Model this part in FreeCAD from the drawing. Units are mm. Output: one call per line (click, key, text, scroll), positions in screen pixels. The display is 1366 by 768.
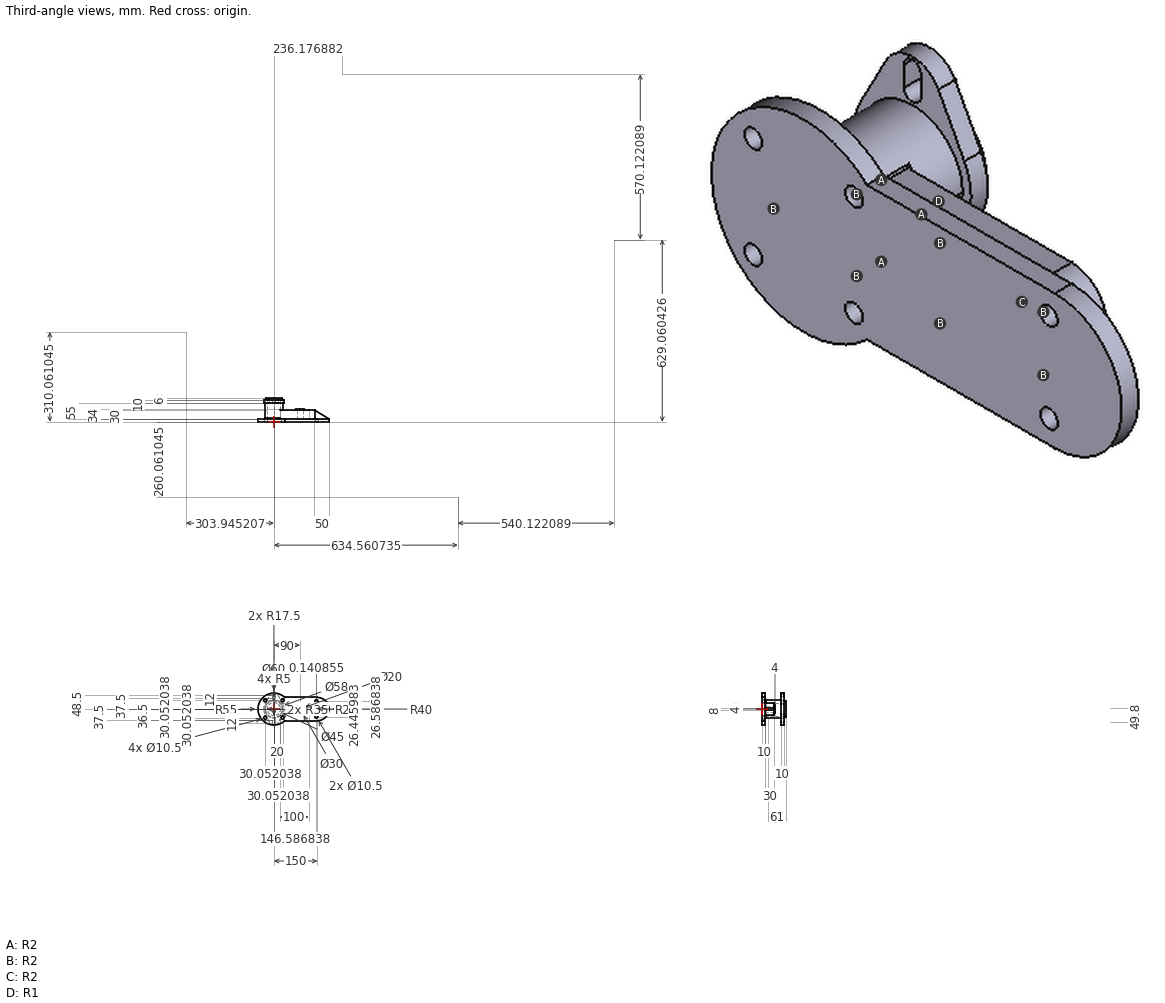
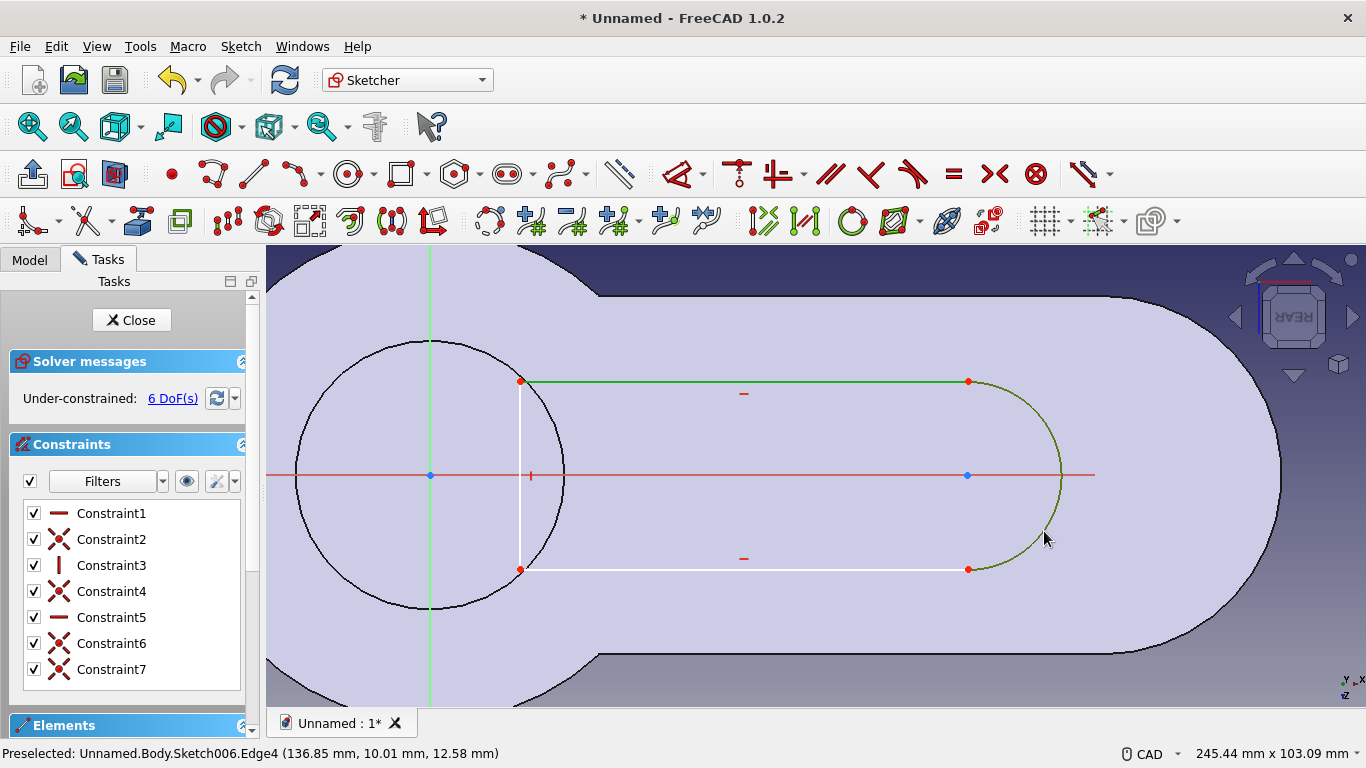
key(t)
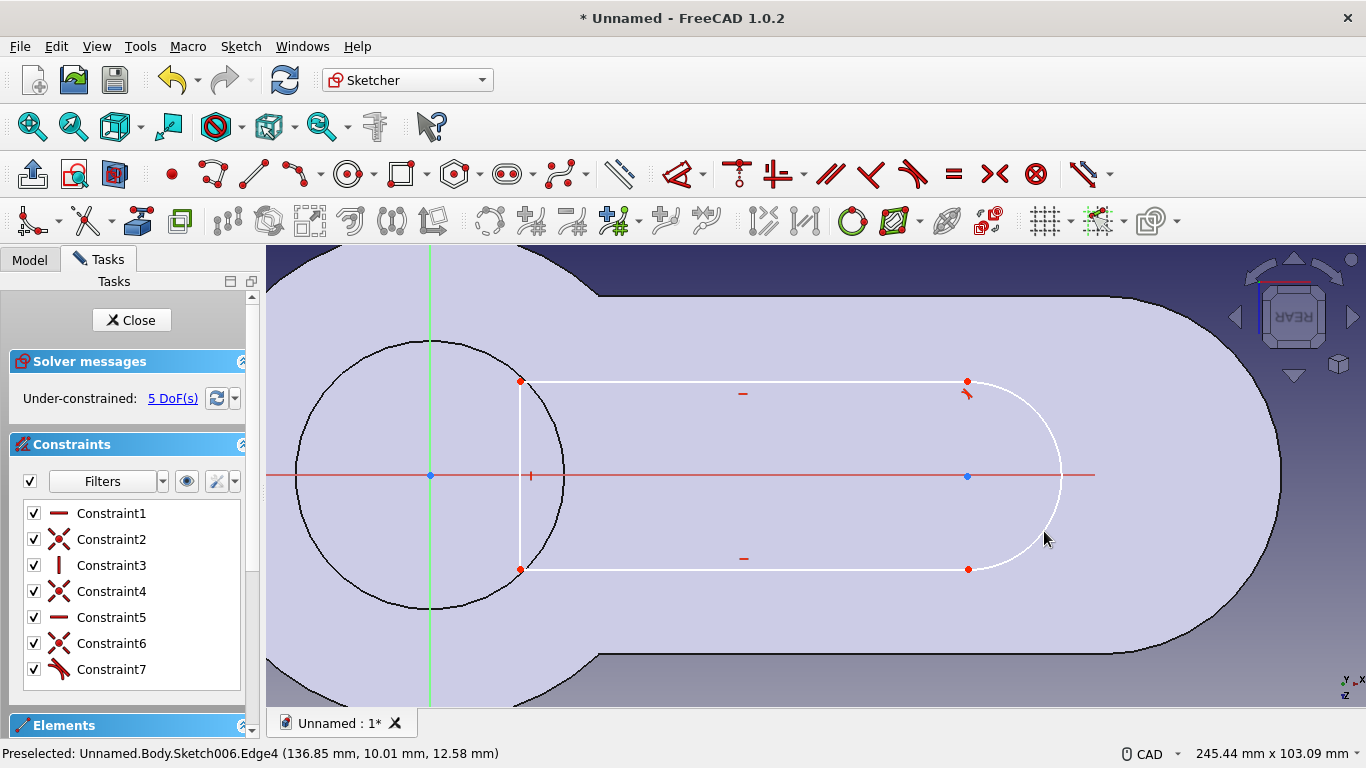
click(654, 570)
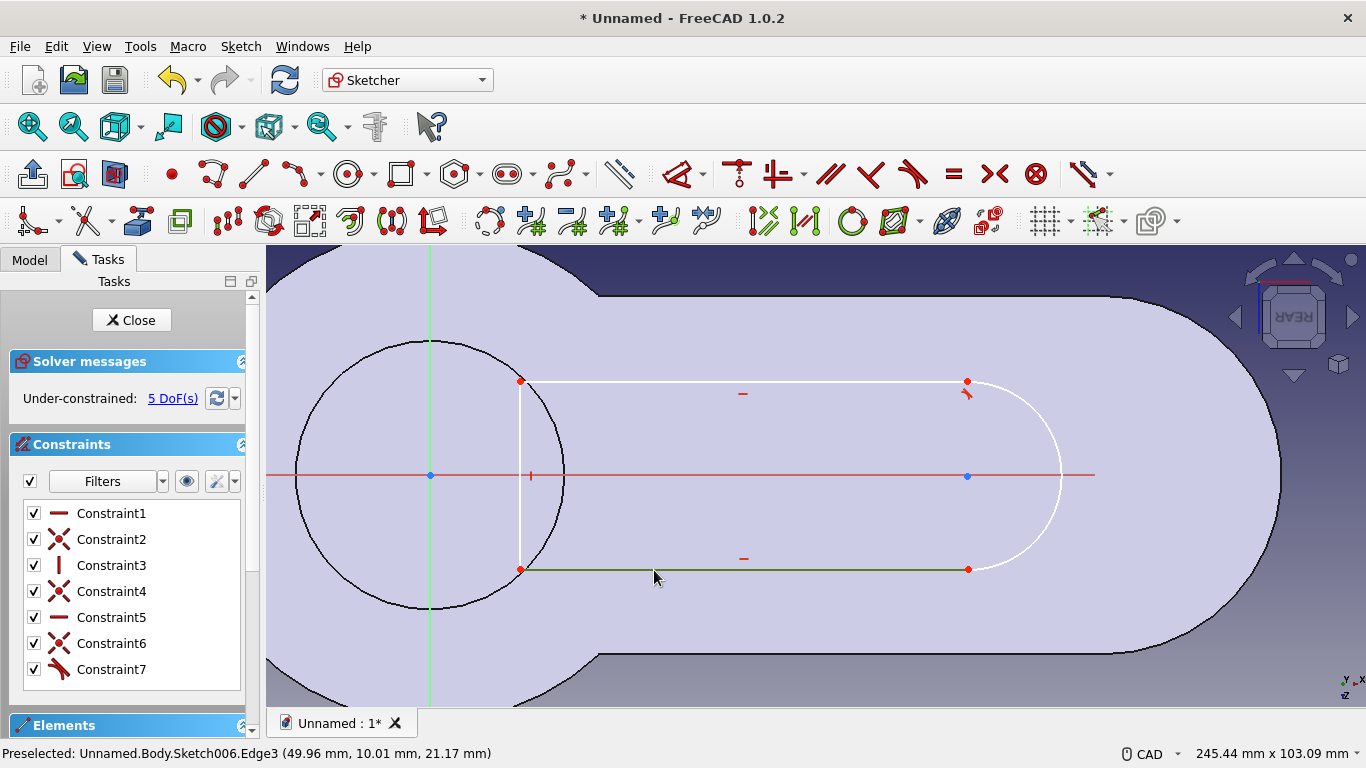
click(1044, 531)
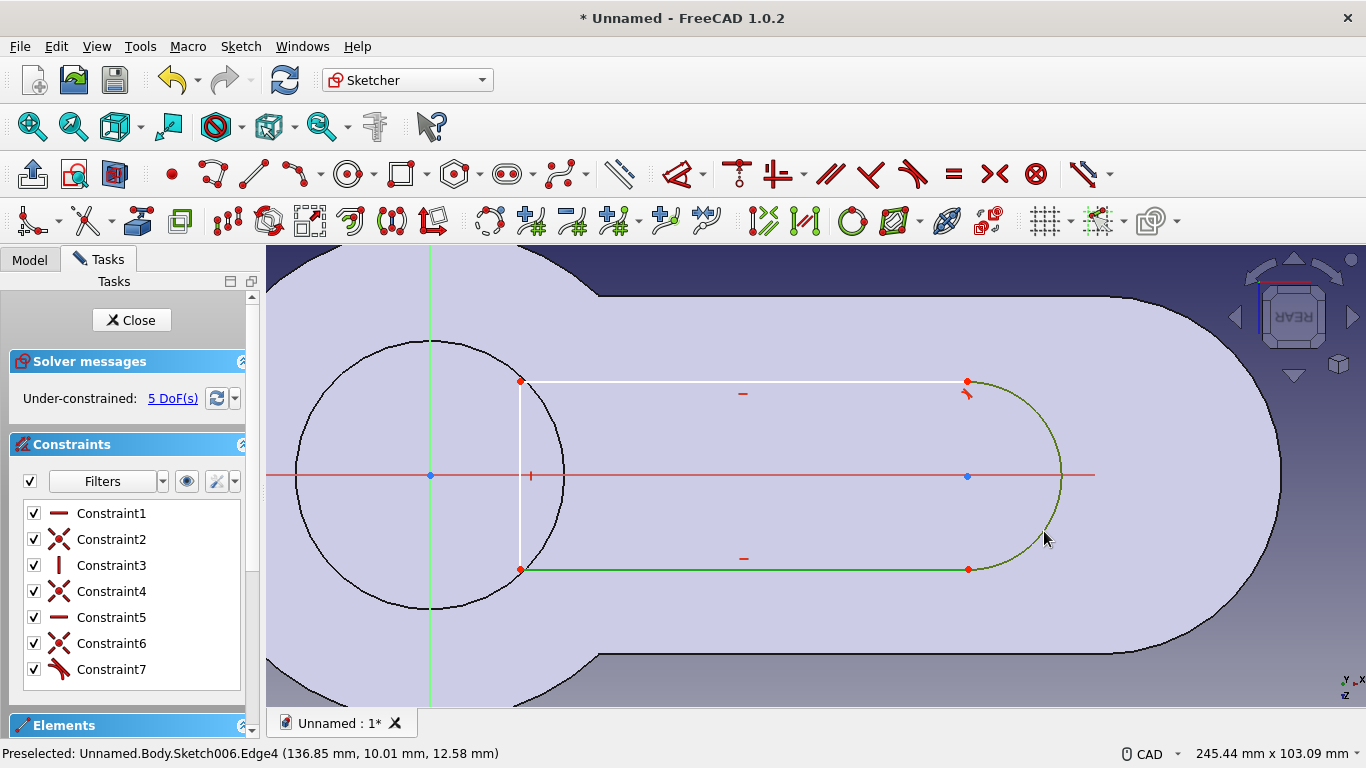
key(t)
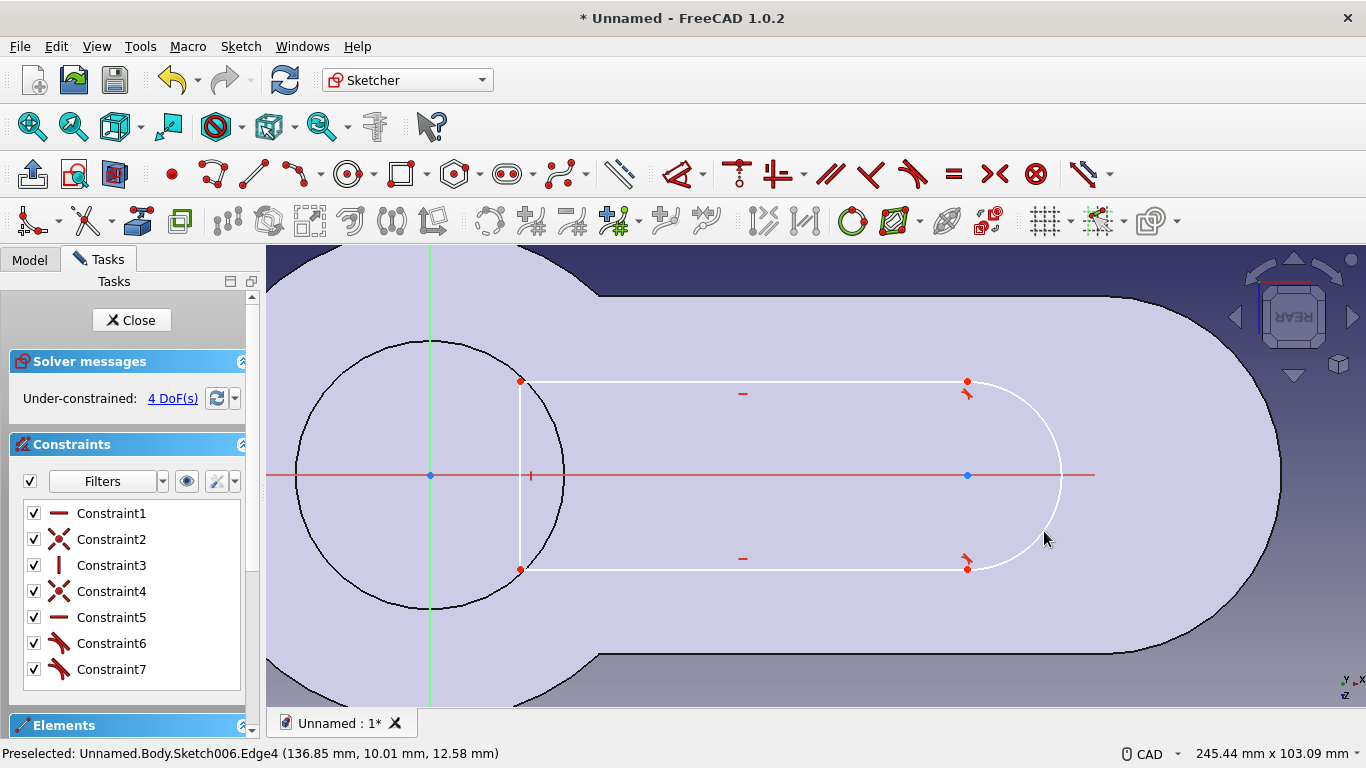
click(968, 476)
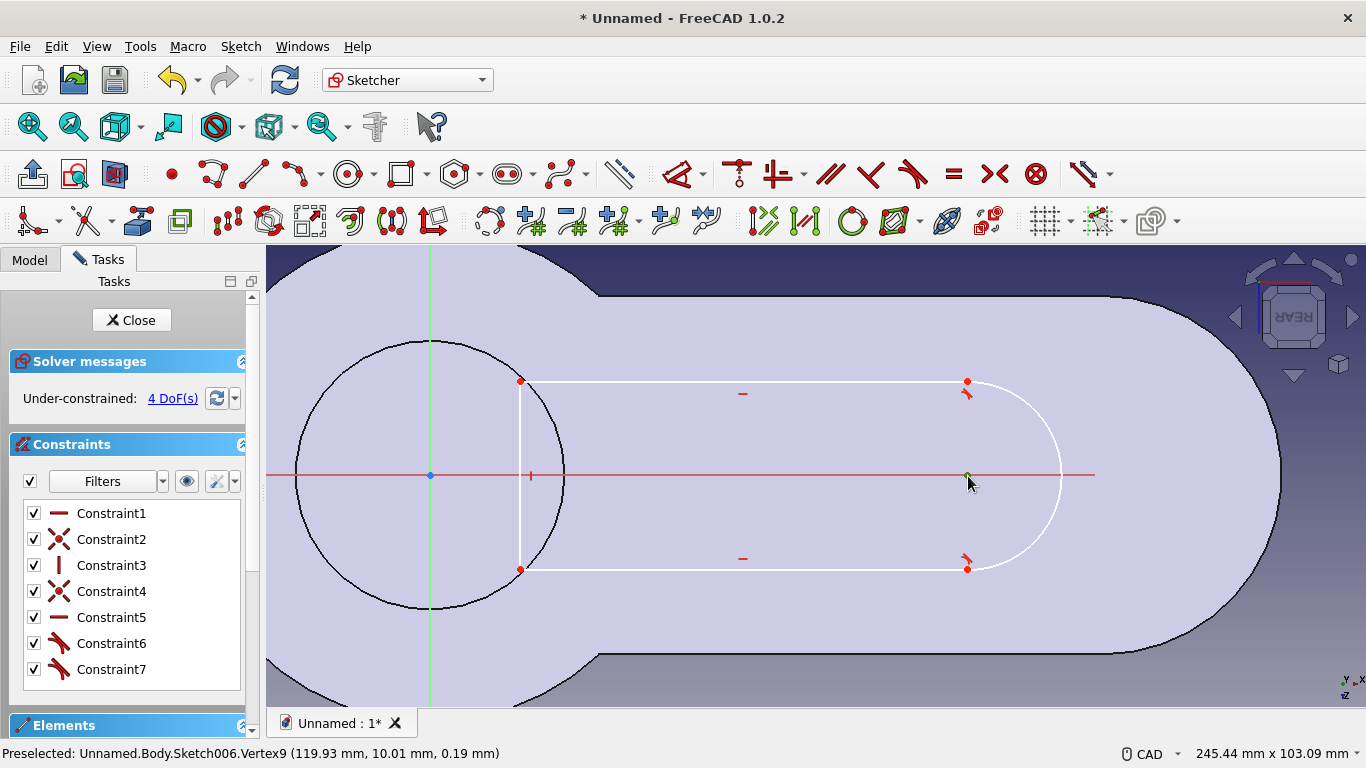
click(359, 475)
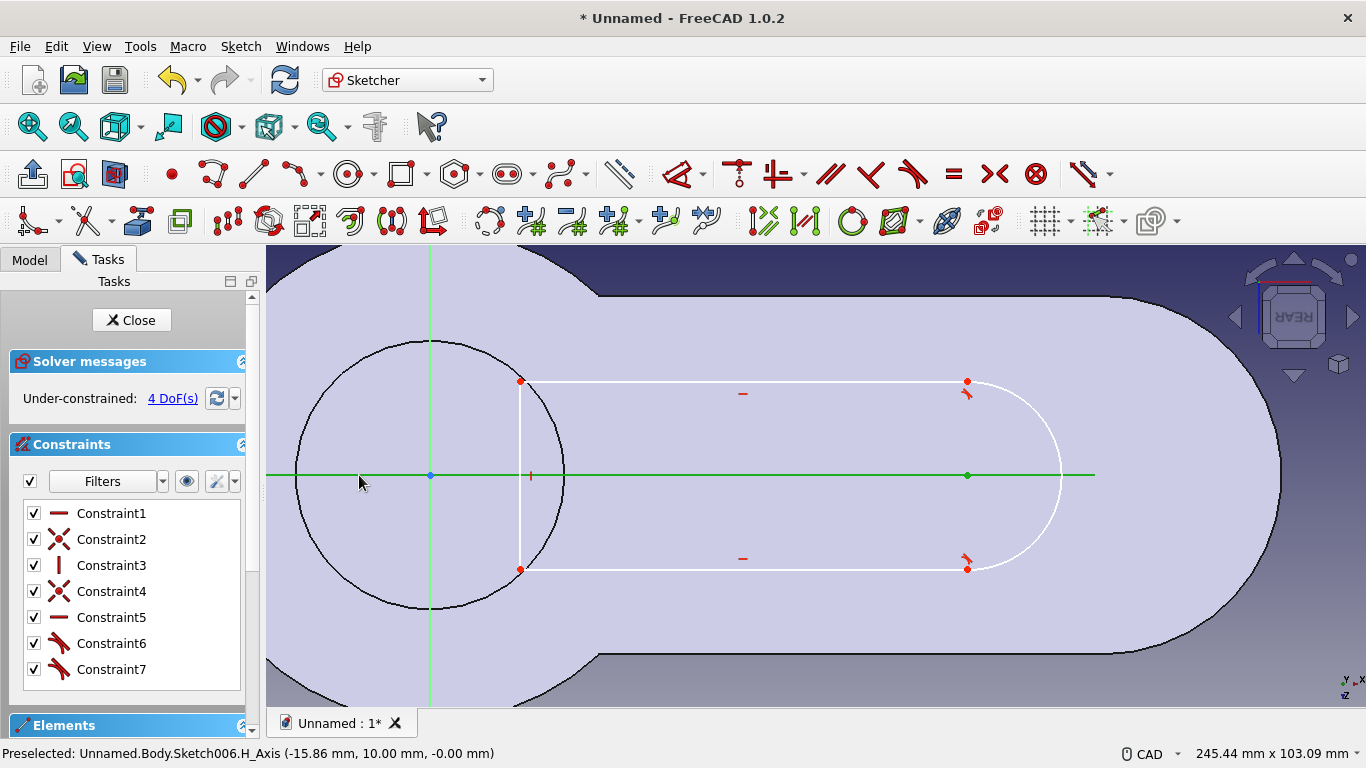
key(c)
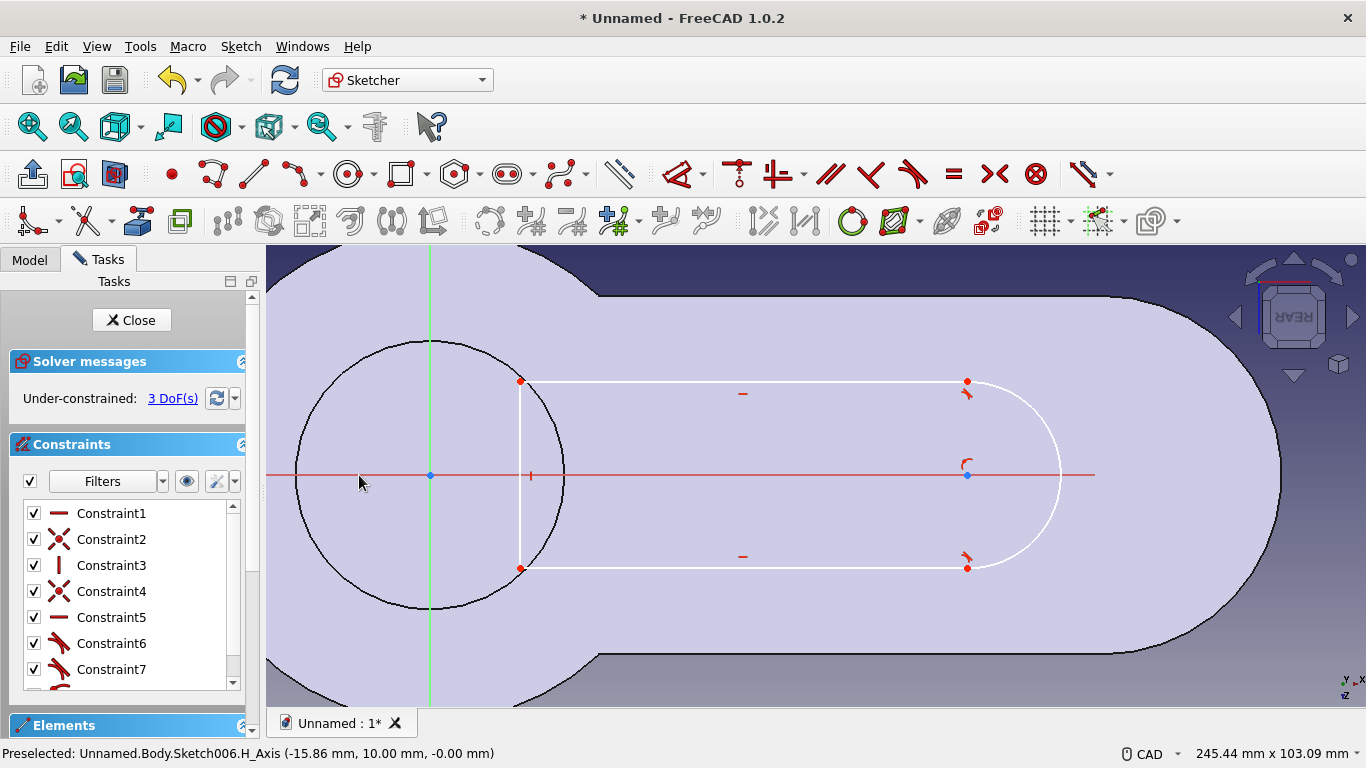
key(d)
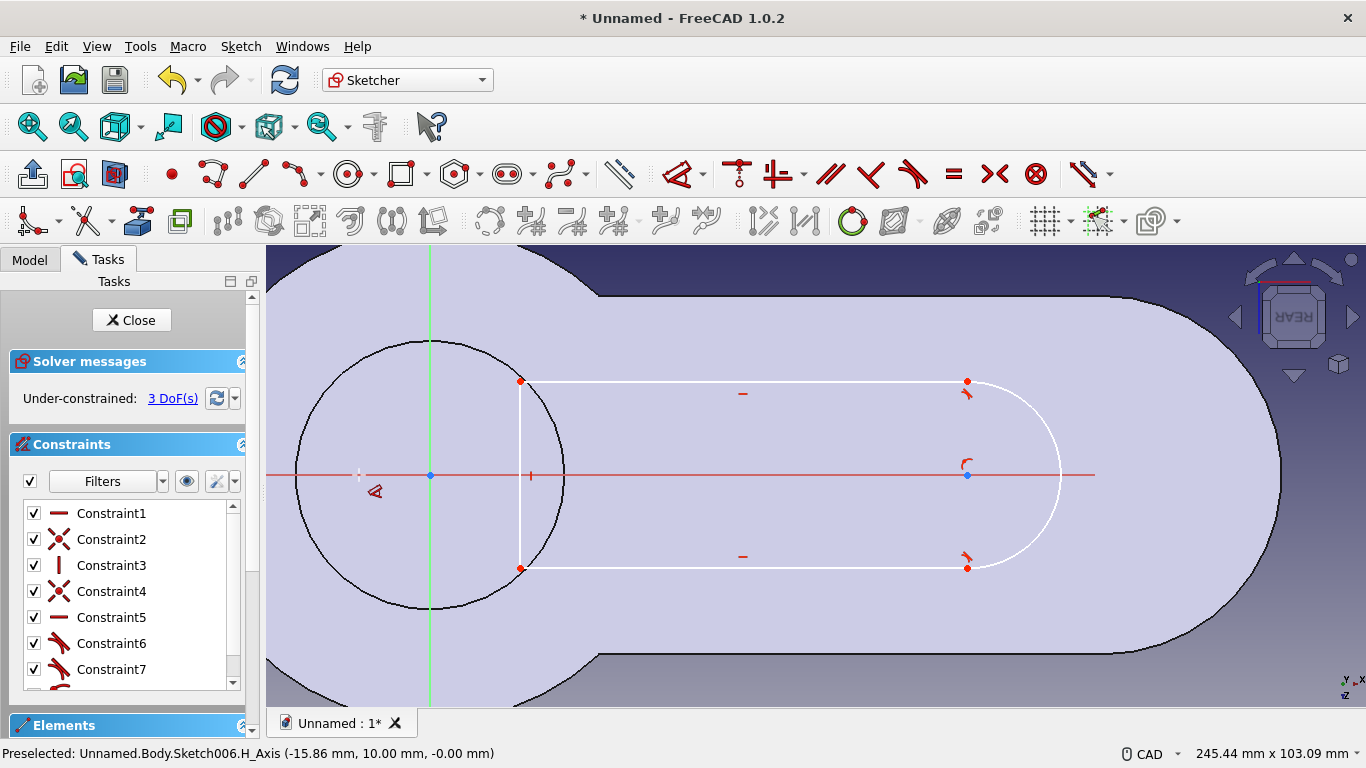
click(1043, 530)
click(1069, 549)